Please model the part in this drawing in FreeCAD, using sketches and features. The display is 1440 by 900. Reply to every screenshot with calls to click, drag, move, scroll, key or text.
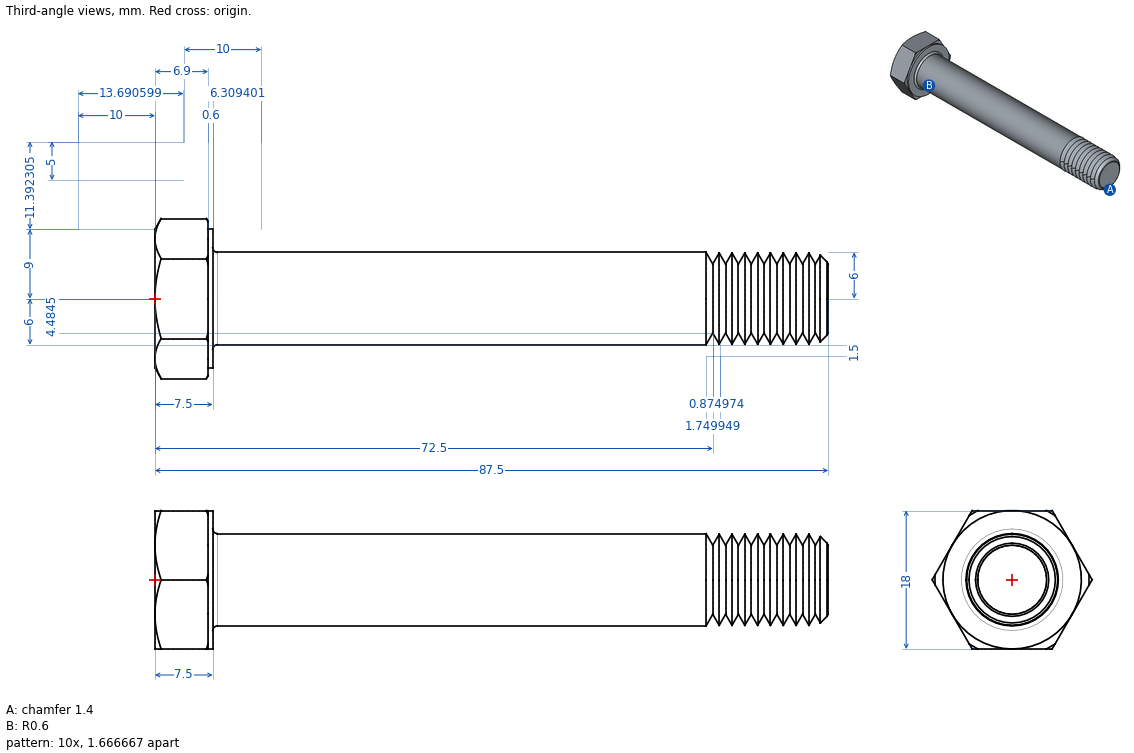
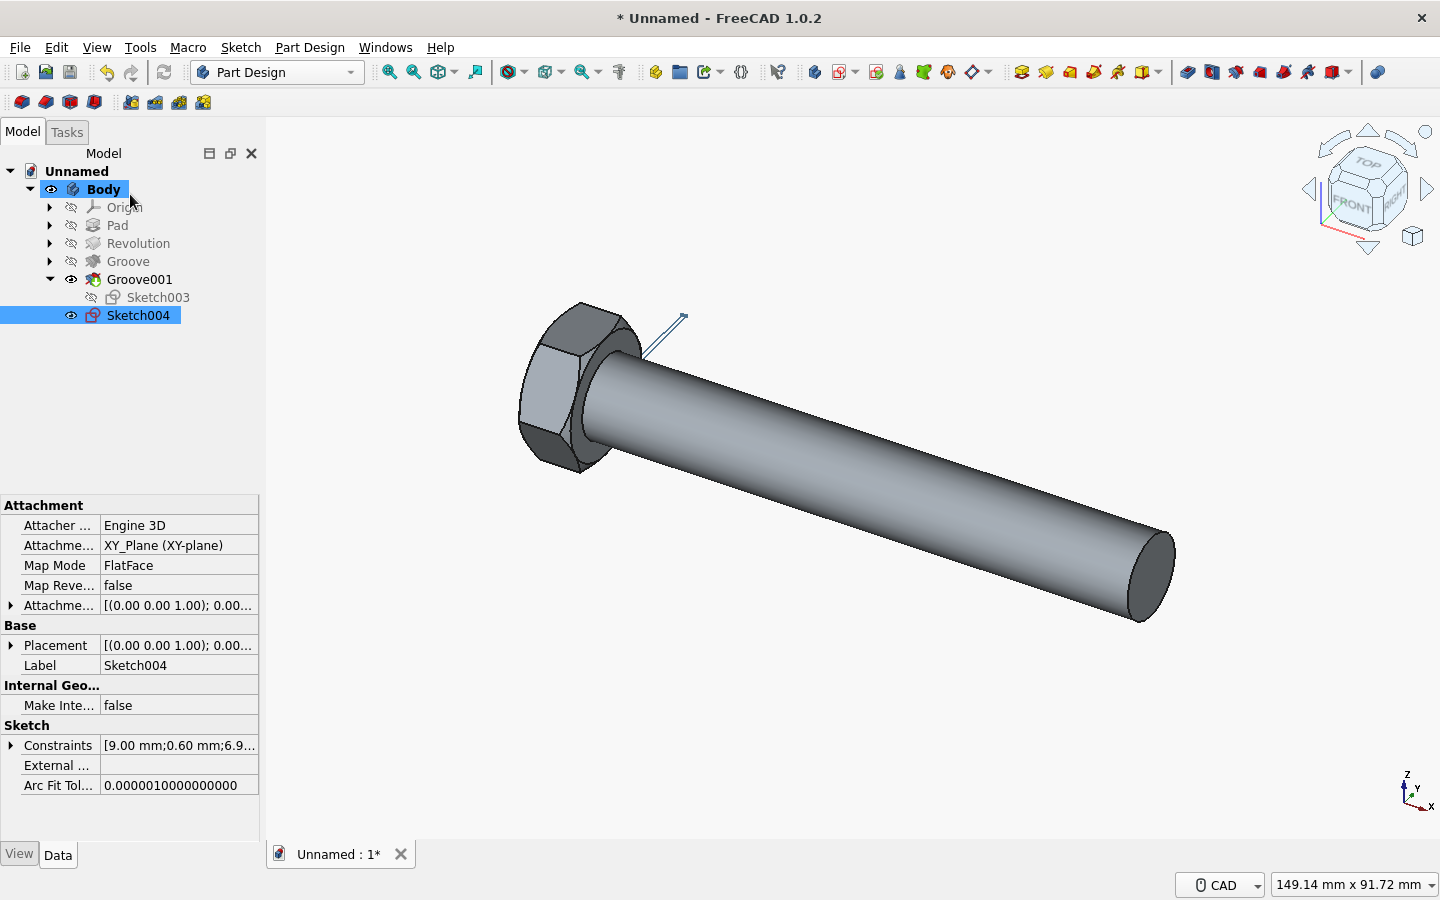
click(1236, 72)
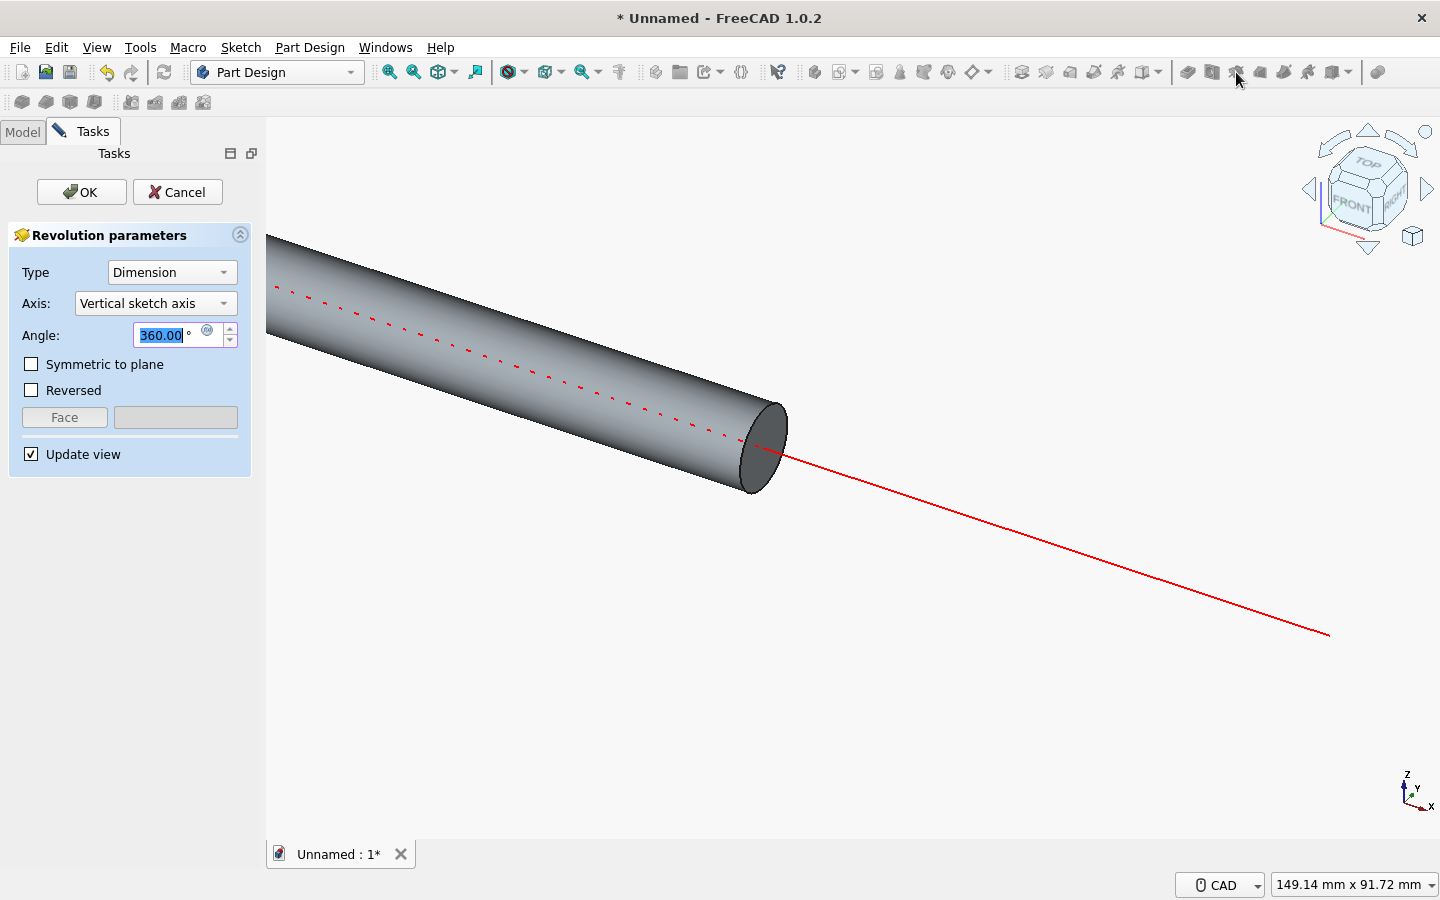
click(156, 304)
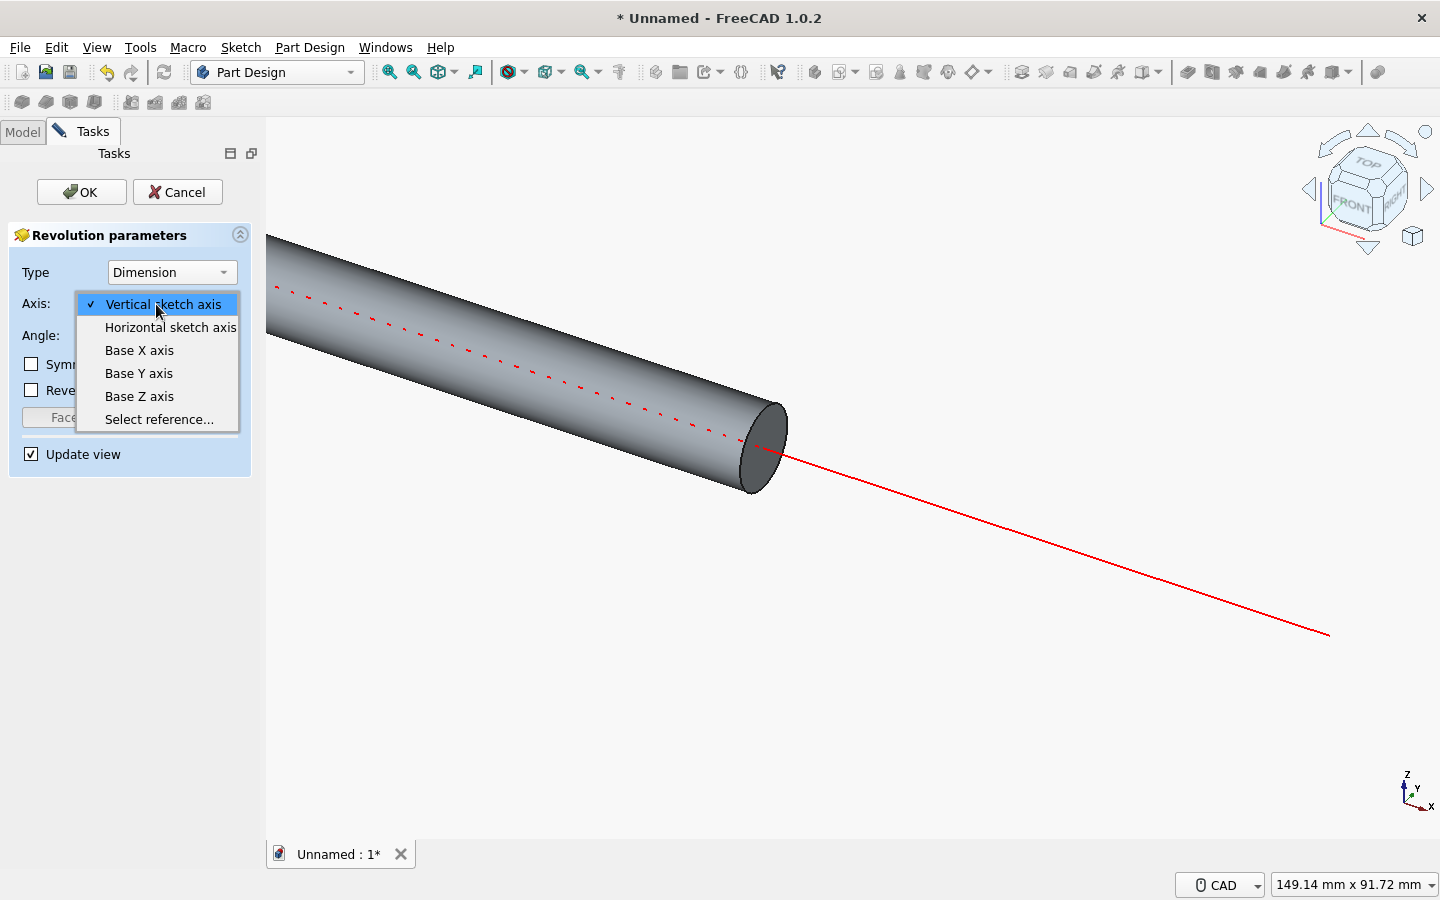
click(156, 328)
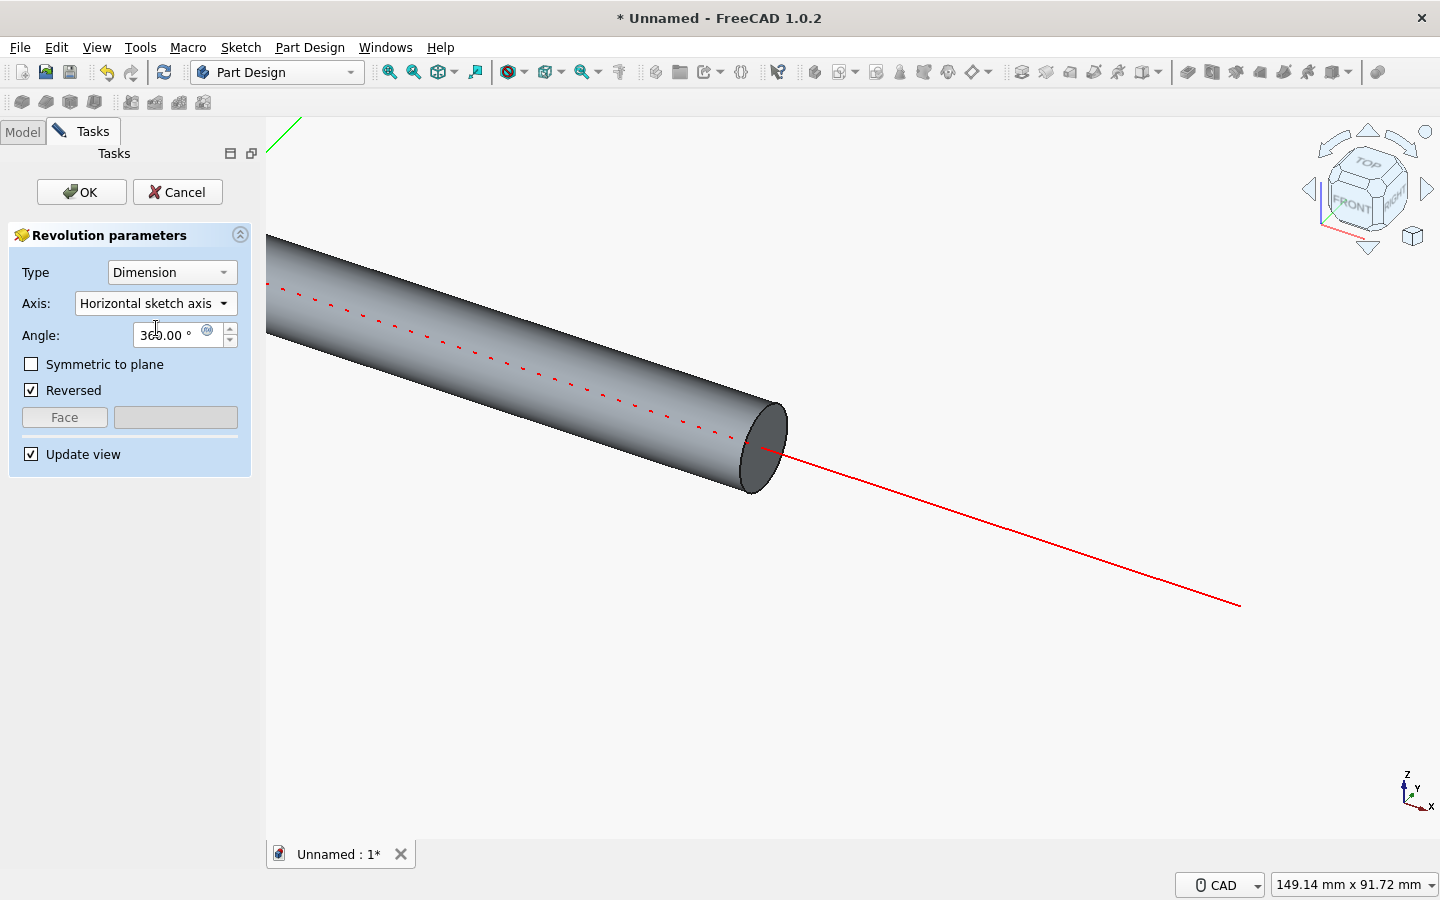
click(82, 192)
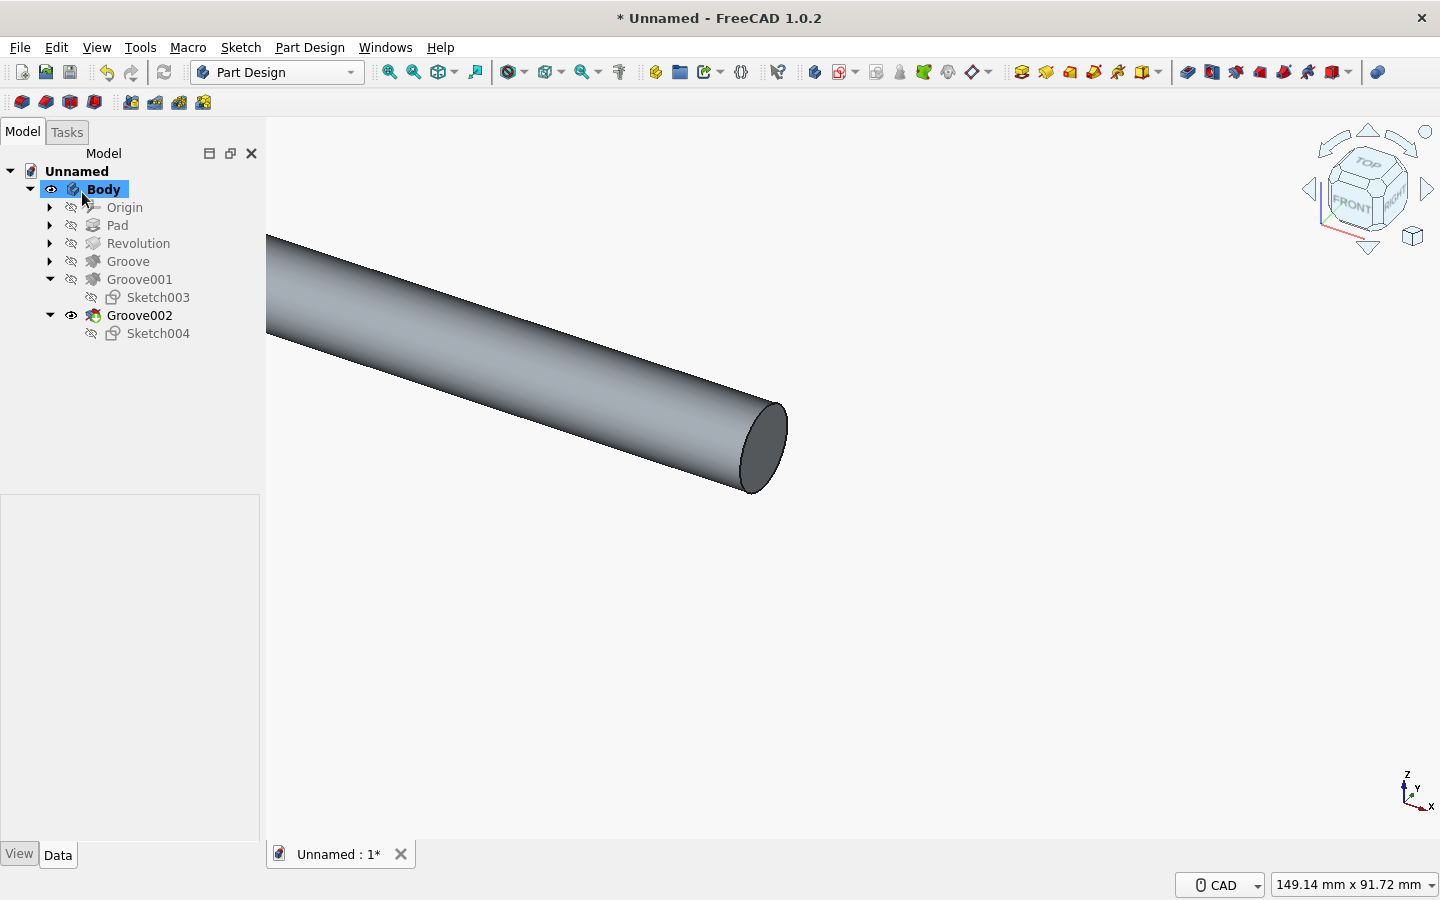
click(390, 72)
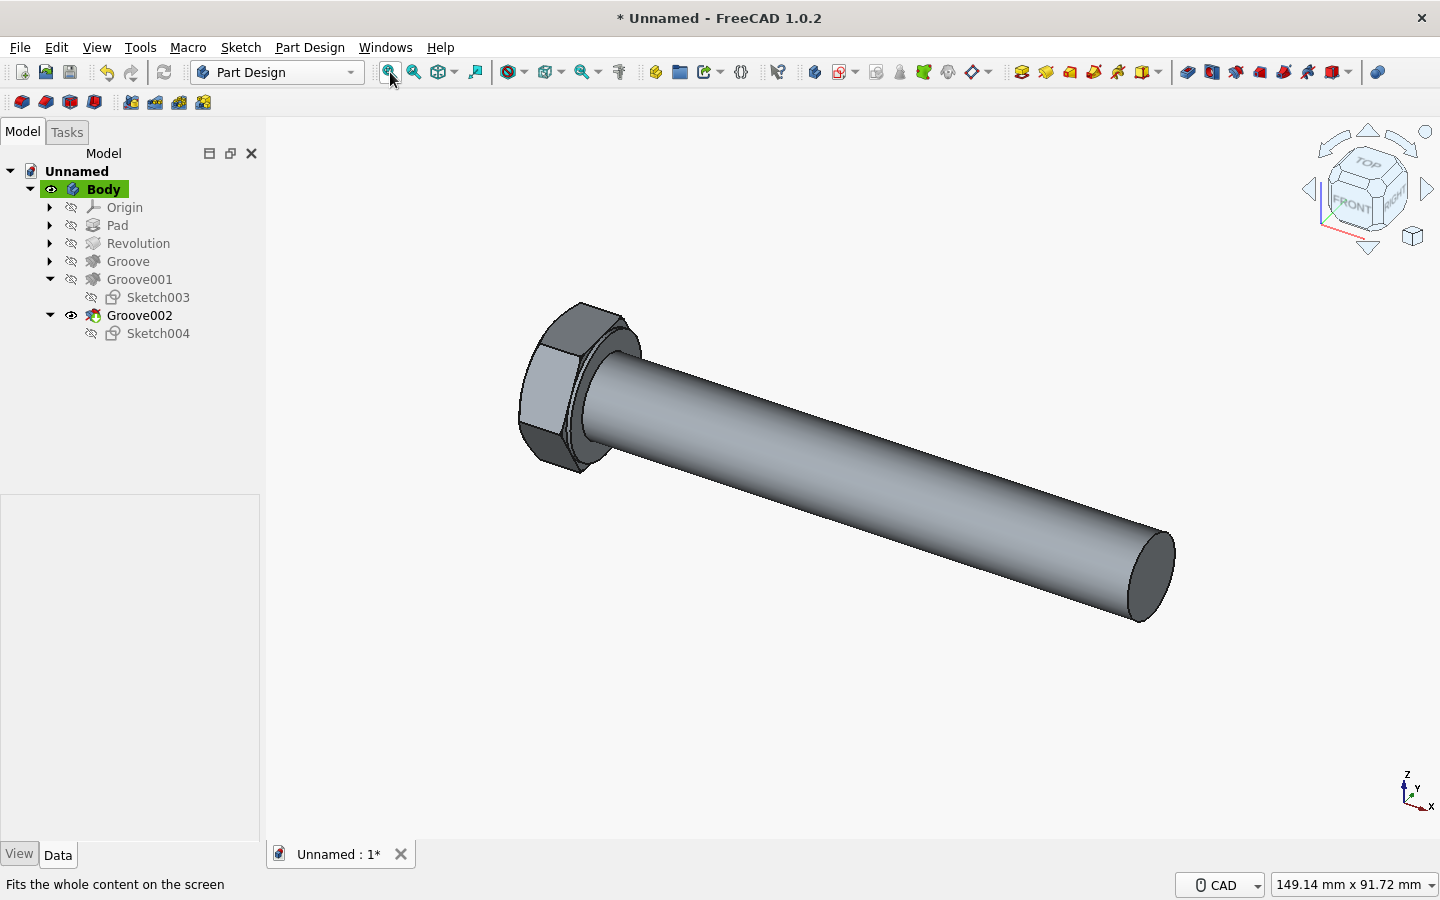
click(1128, 599)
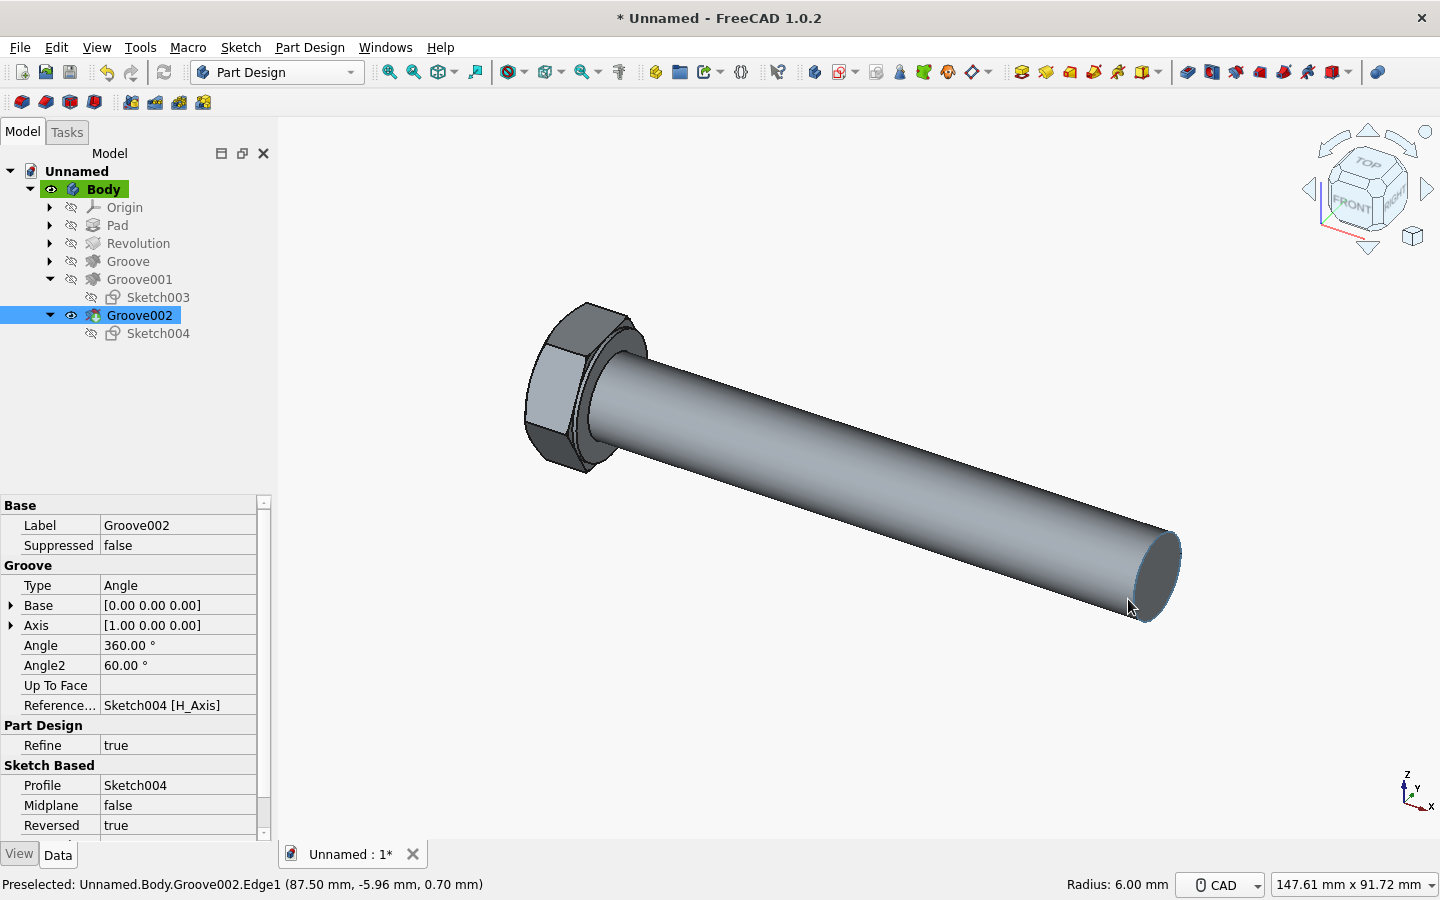
click(46, 102)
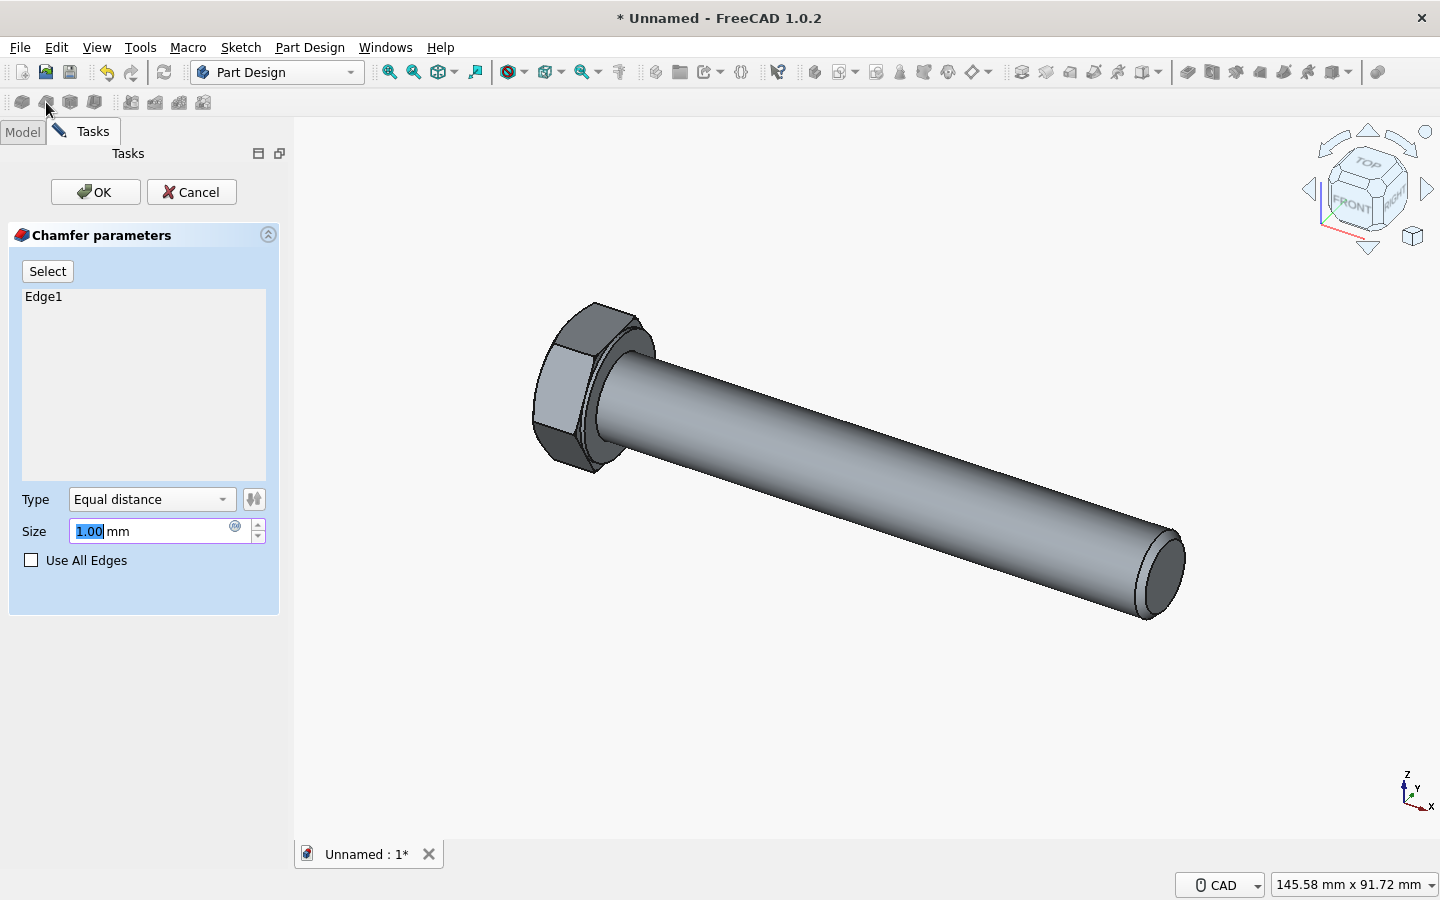
text(1.4)
key(Tab)